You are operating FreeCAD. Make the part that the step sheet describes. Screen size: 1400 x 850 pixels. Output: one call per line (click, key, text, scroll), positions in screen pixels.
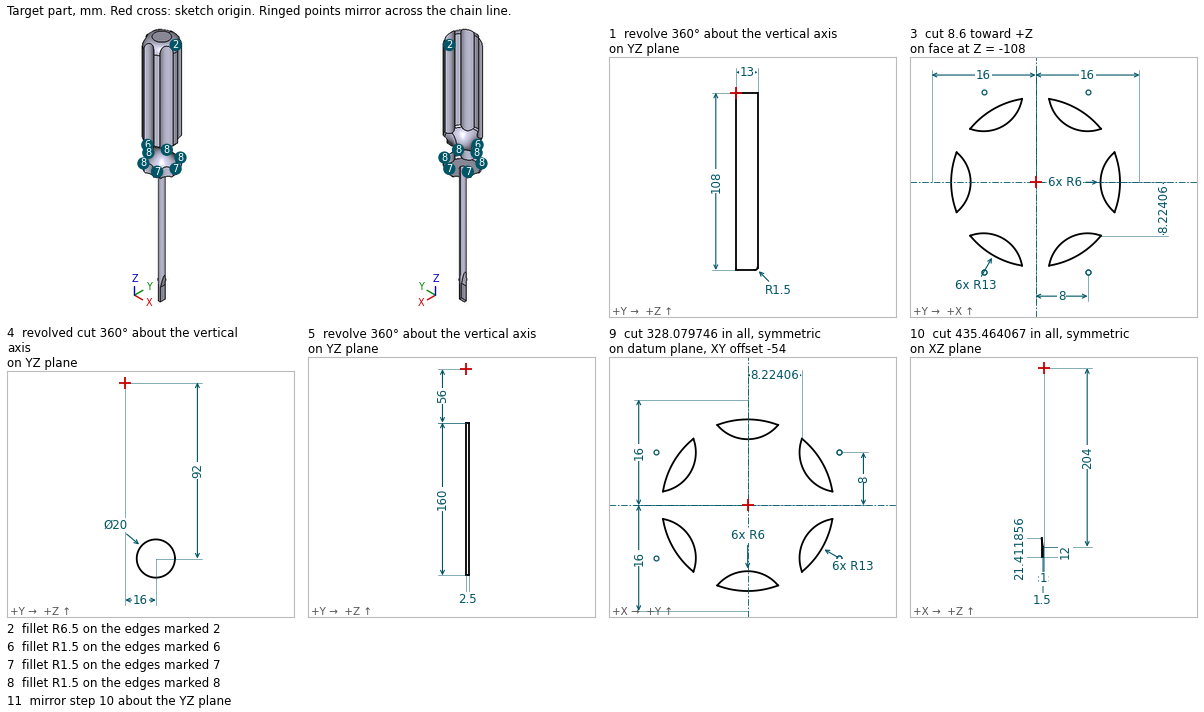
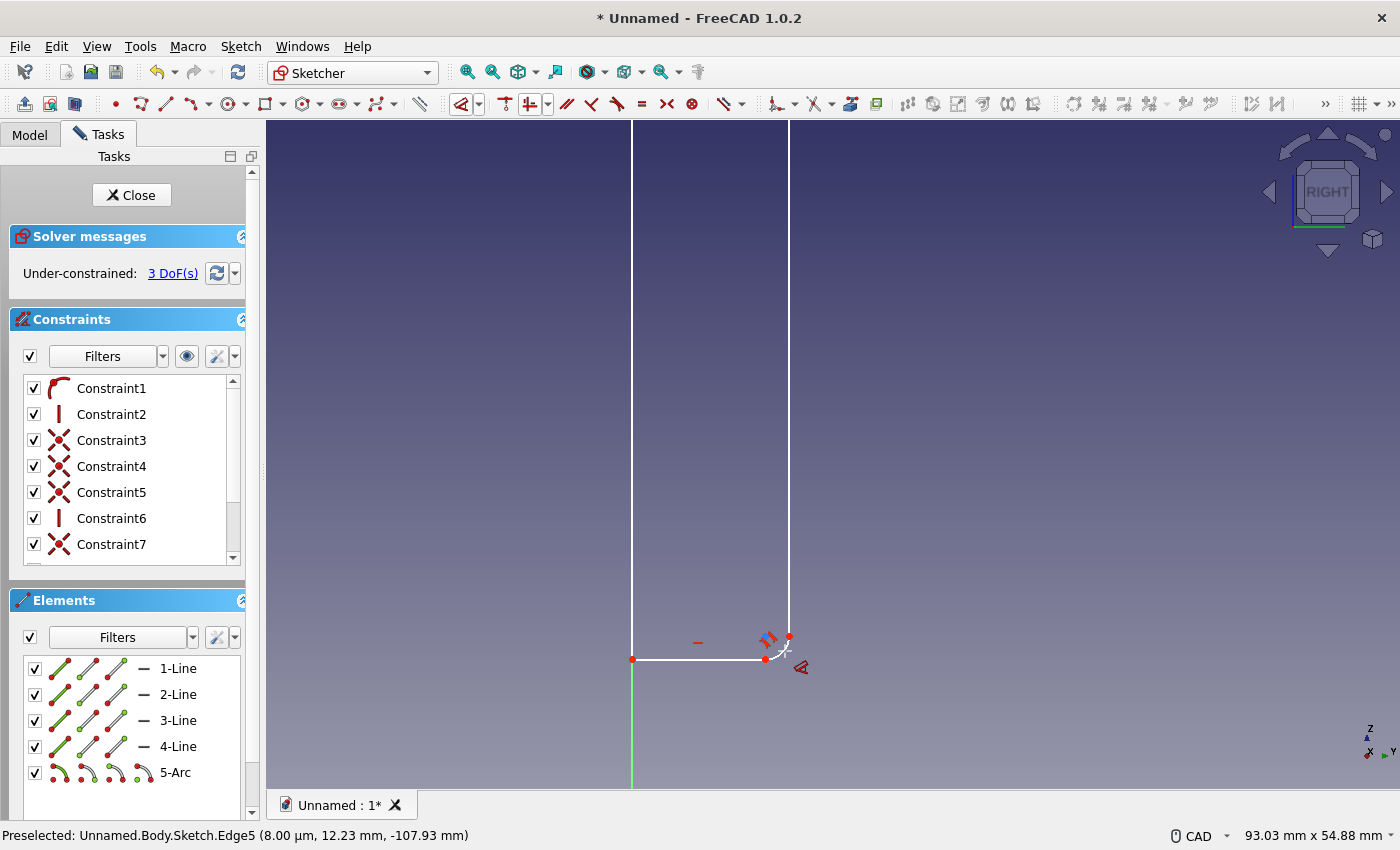
scroll(776, 657, up, 4)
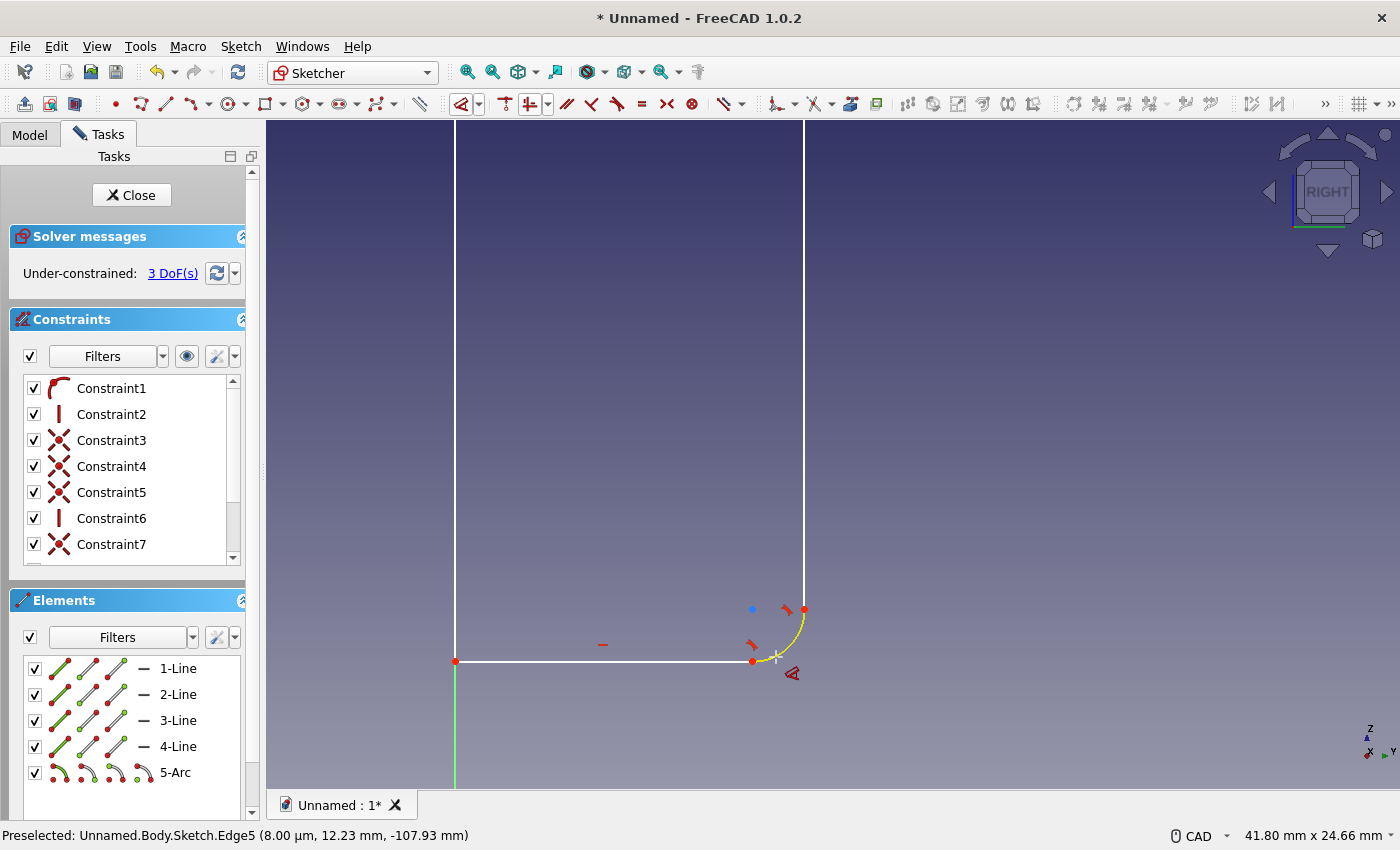
click(776, 656)
click(790, 685)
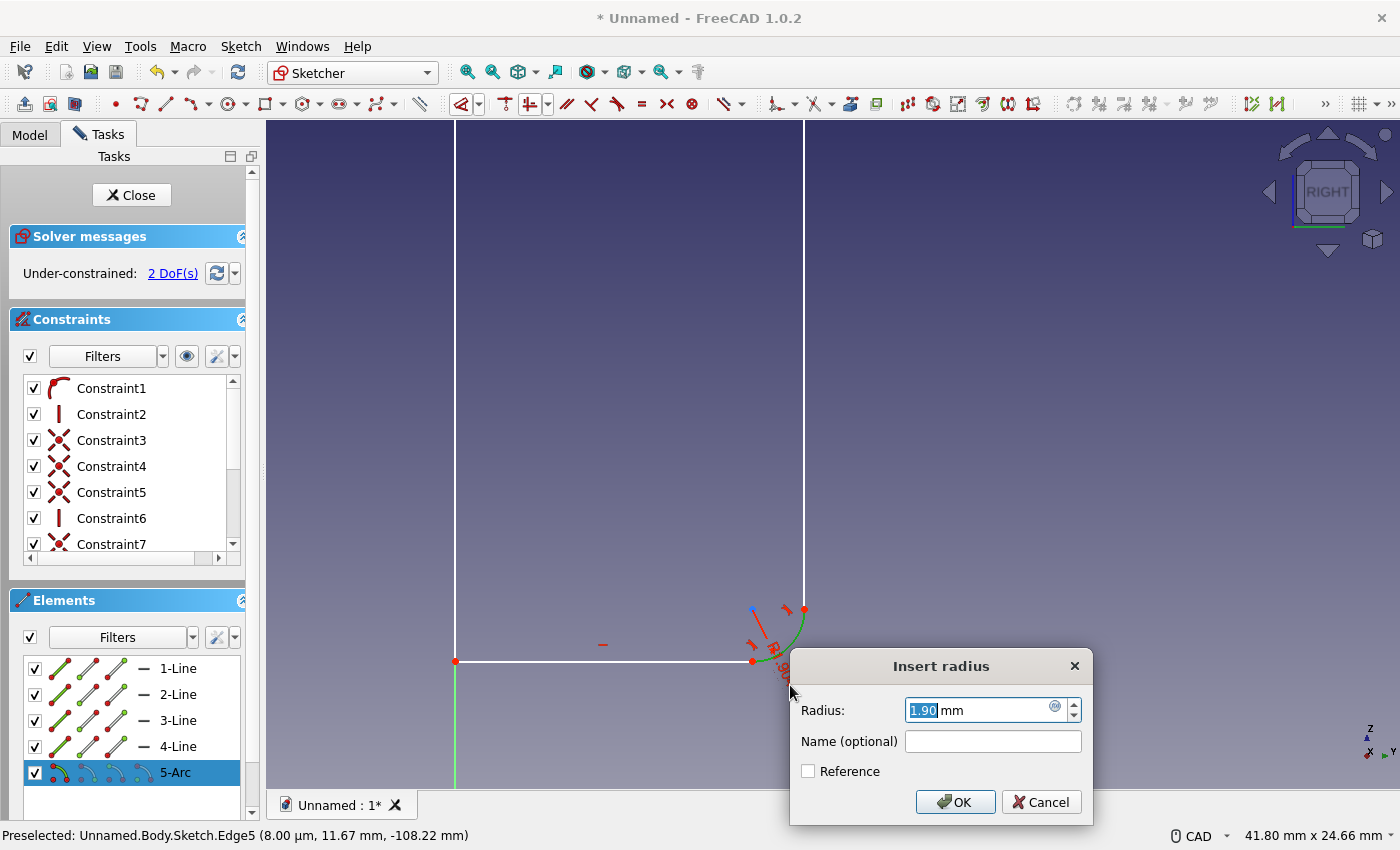
text(1.5)
key(Return)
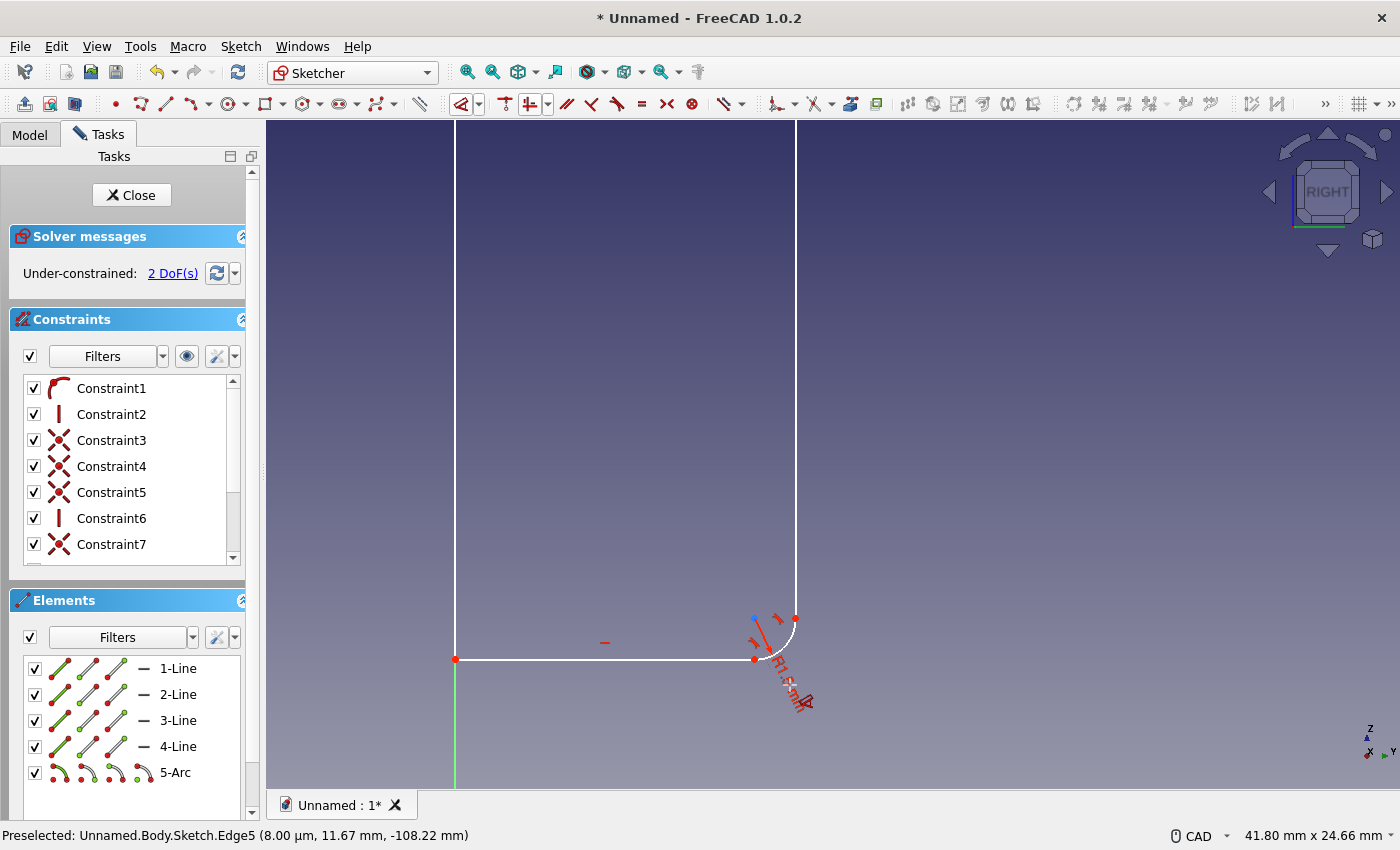
scroll(785, 653, down, 10)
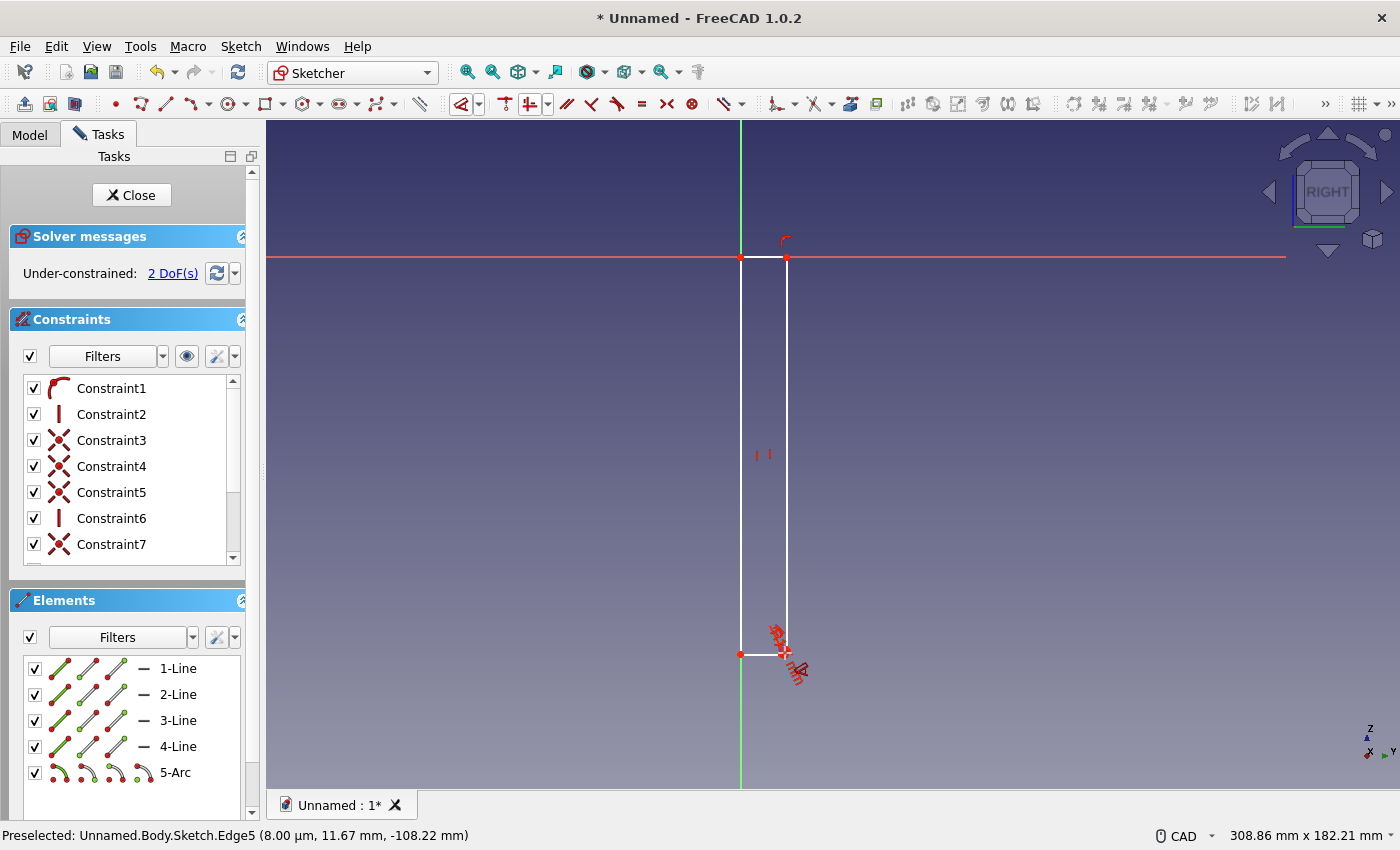
click(773, 257)
click(764, 223)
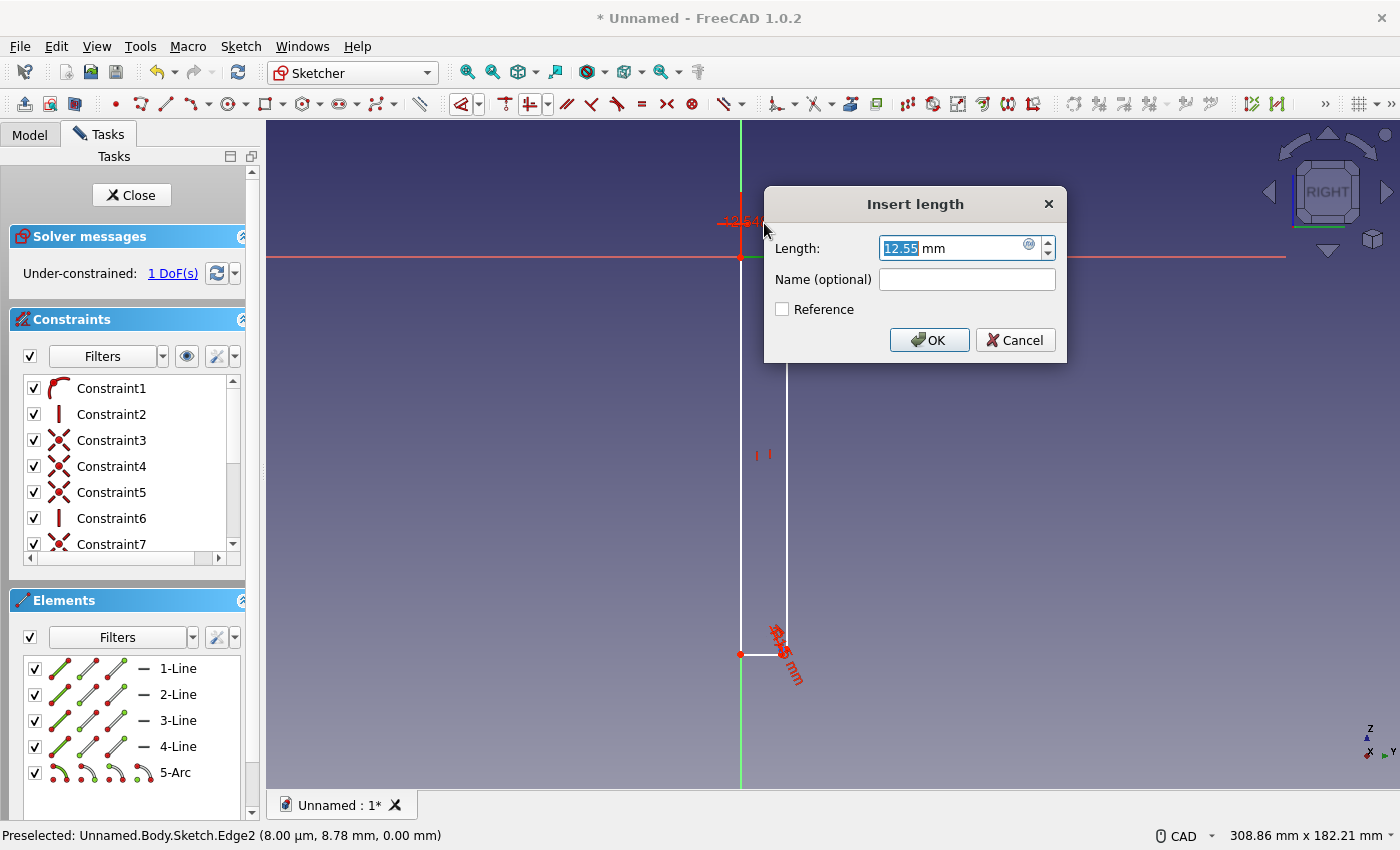
text(13)
key(Return)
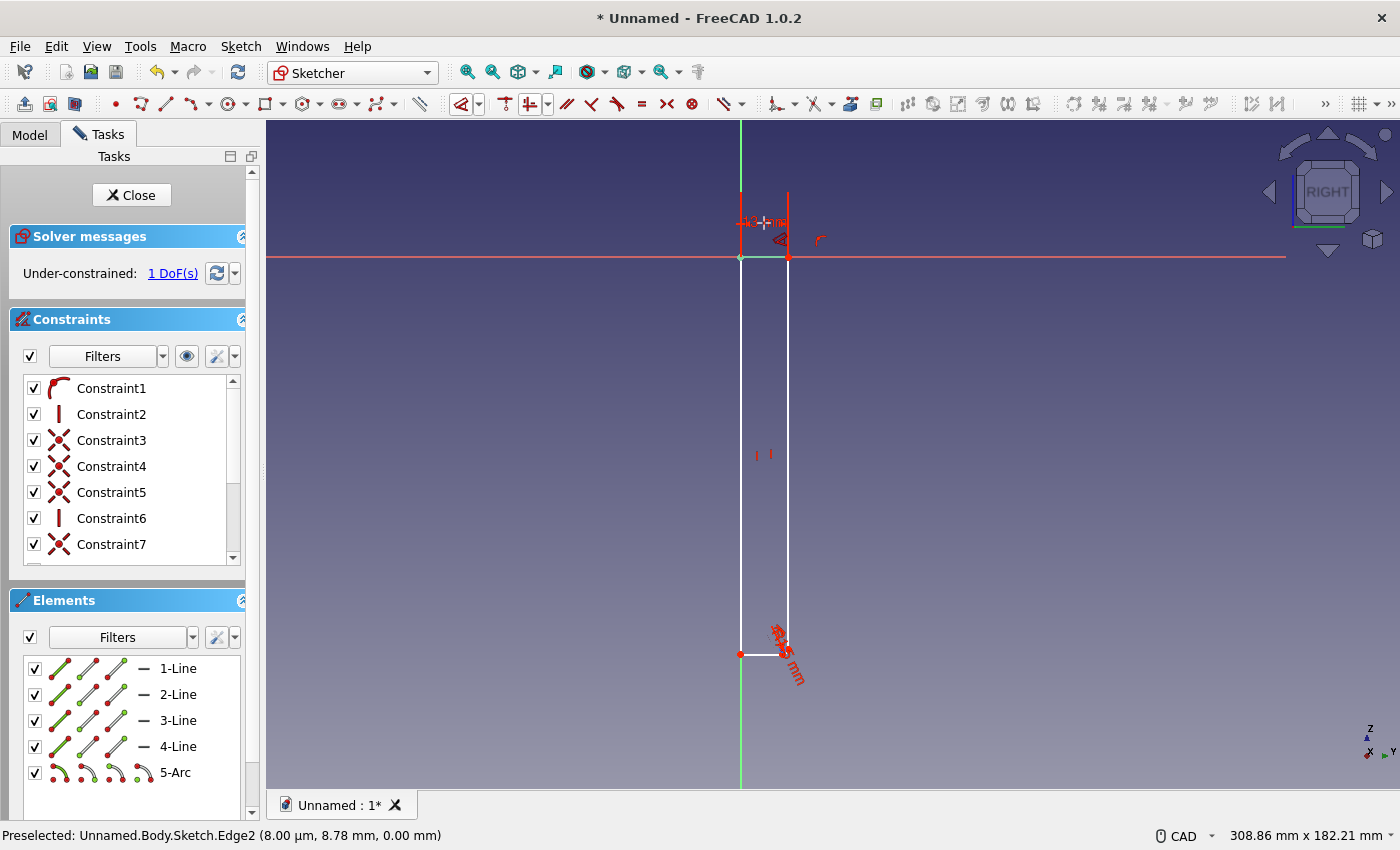
click(741, 376)
click(707, 456)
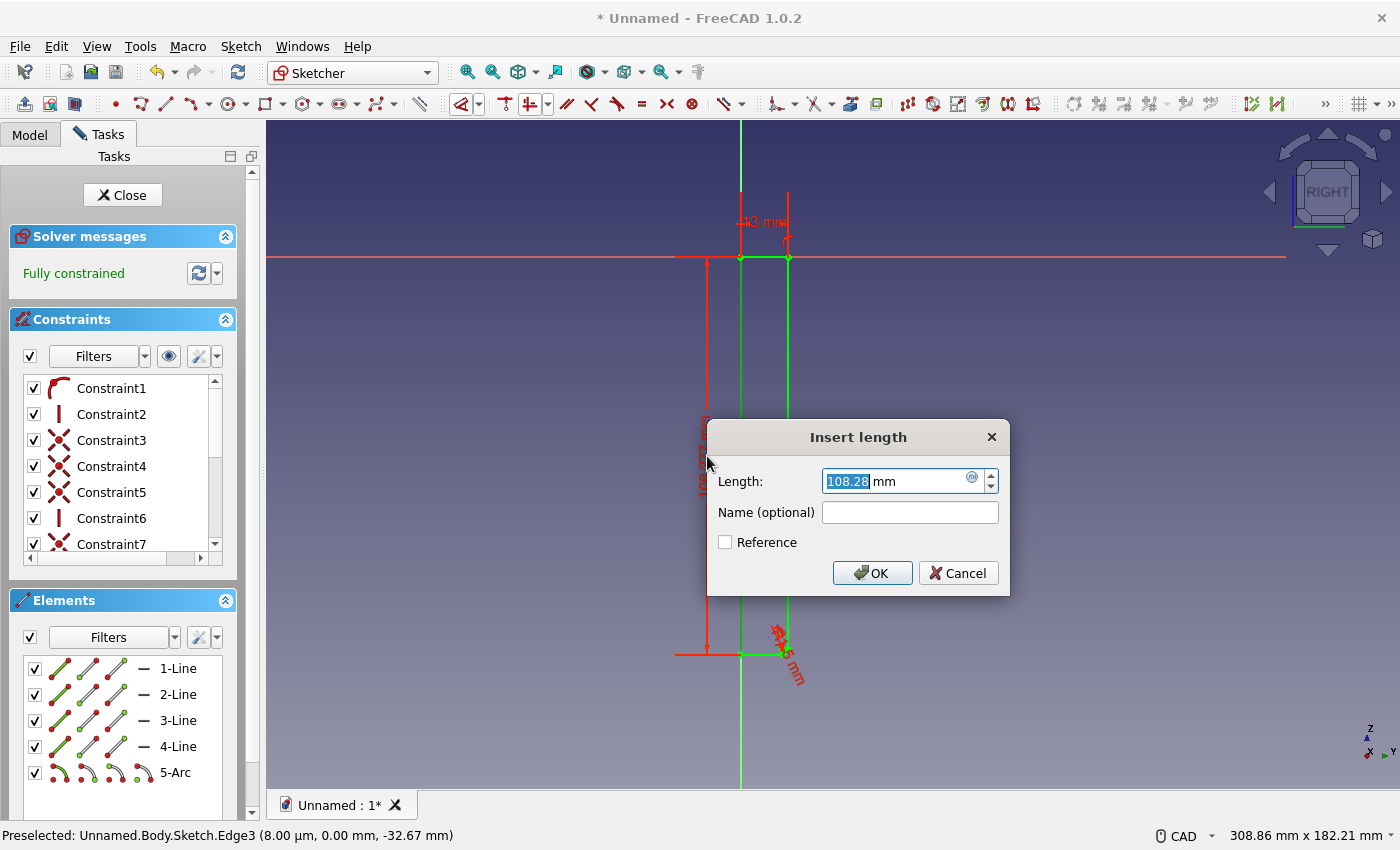
text(108)
key(Return)
key(Escape)